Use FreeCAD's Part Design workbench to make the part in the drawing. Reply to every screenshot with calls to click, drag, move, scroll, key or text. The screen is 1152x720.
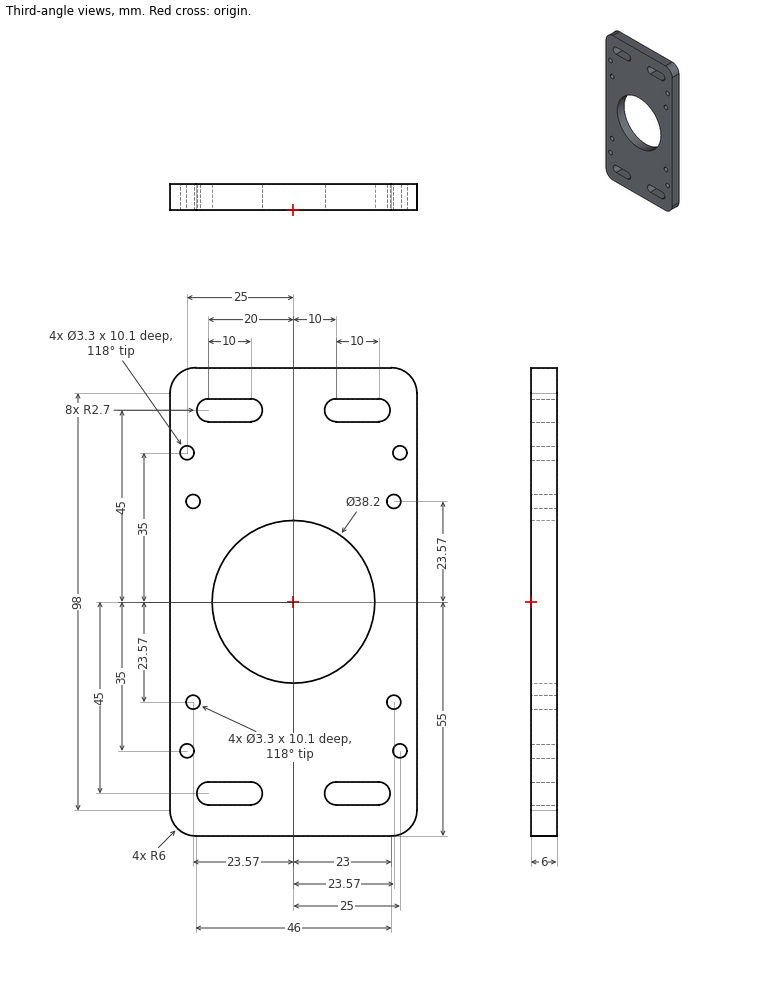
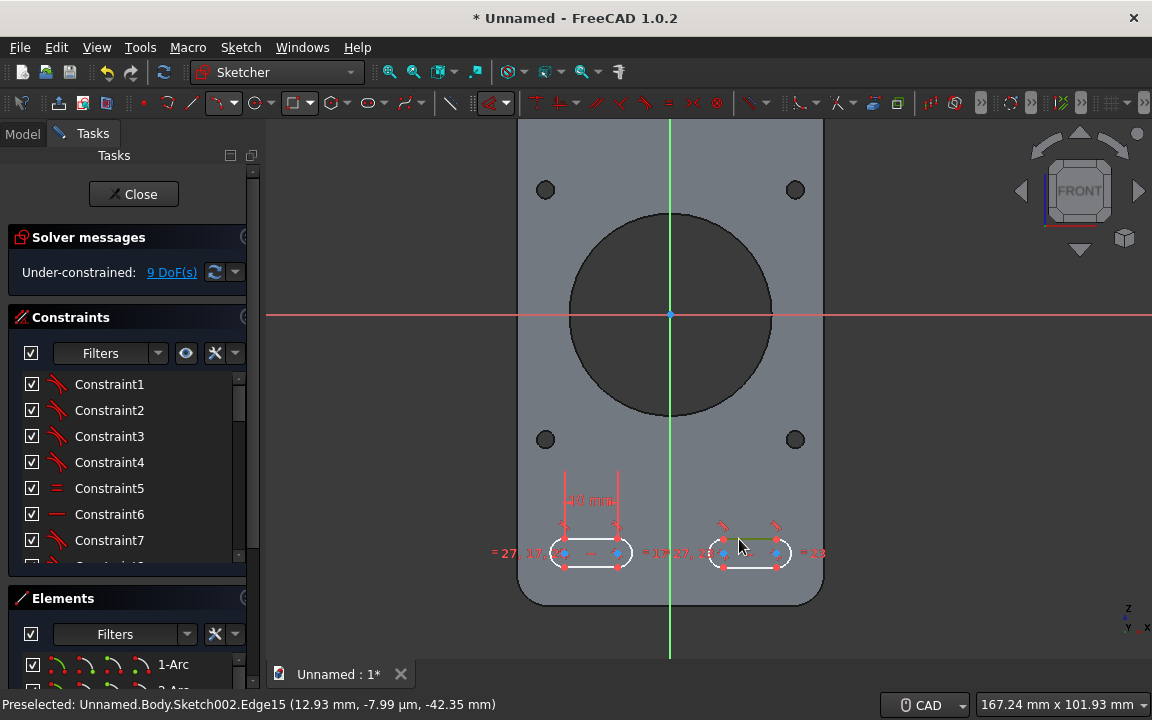
key(l)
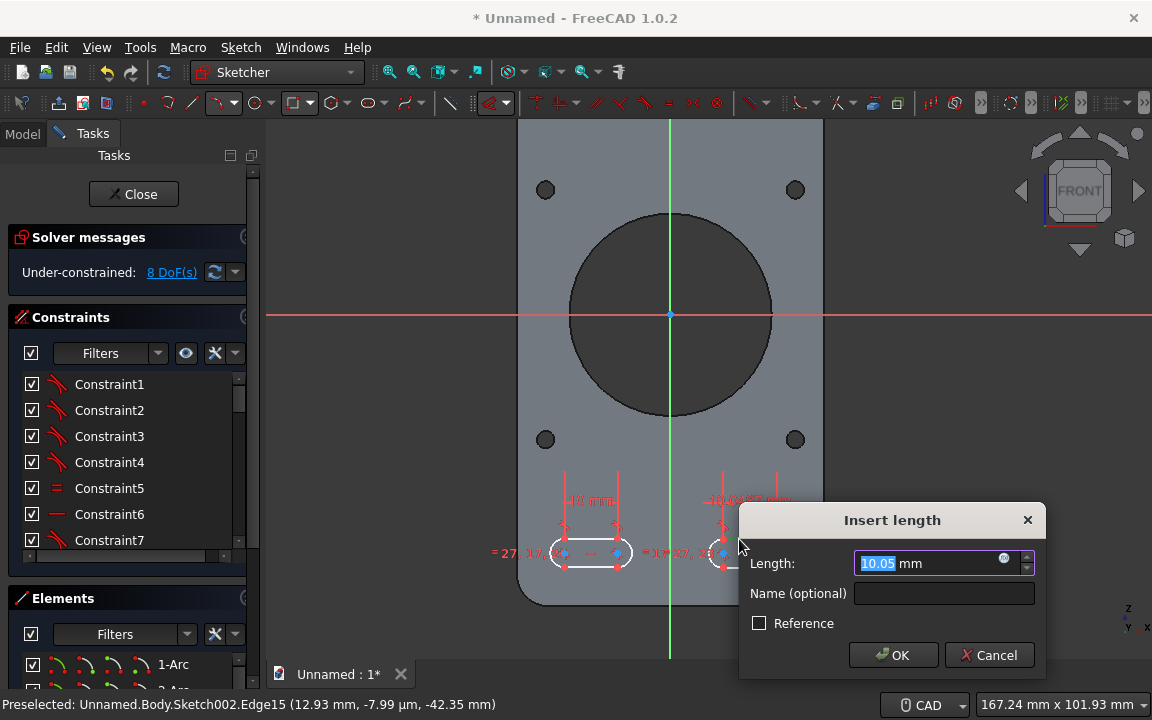
text(10)
key(Return)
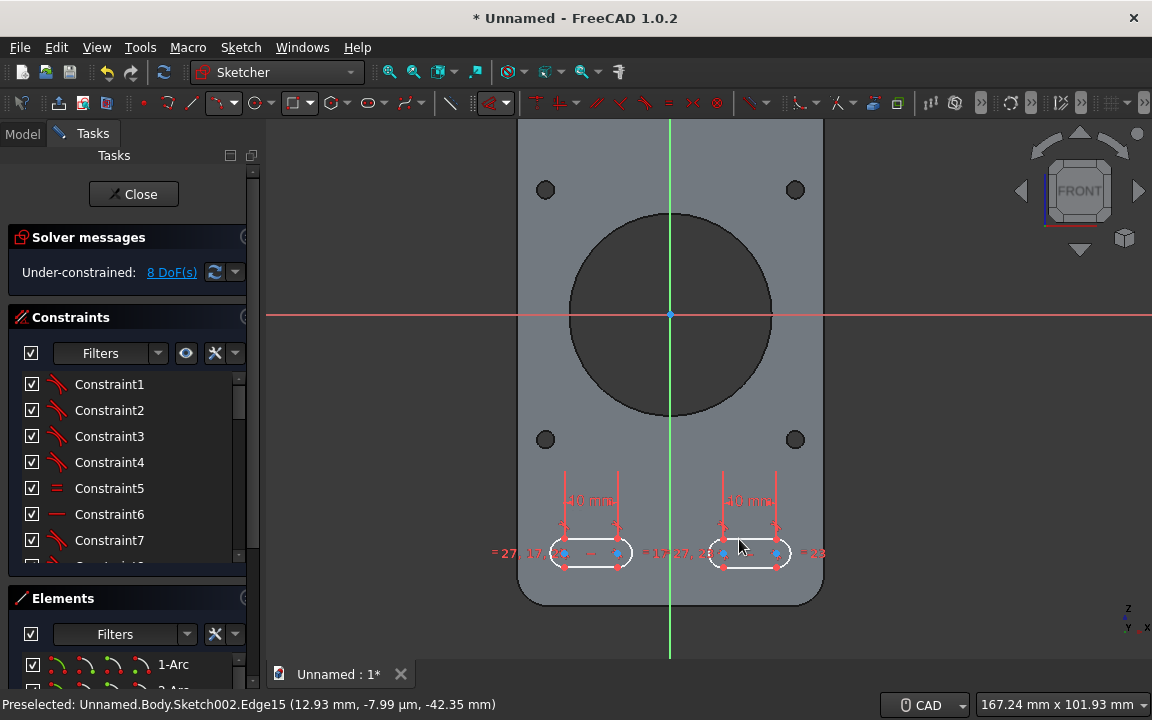
scroll(580, 540, down, 2)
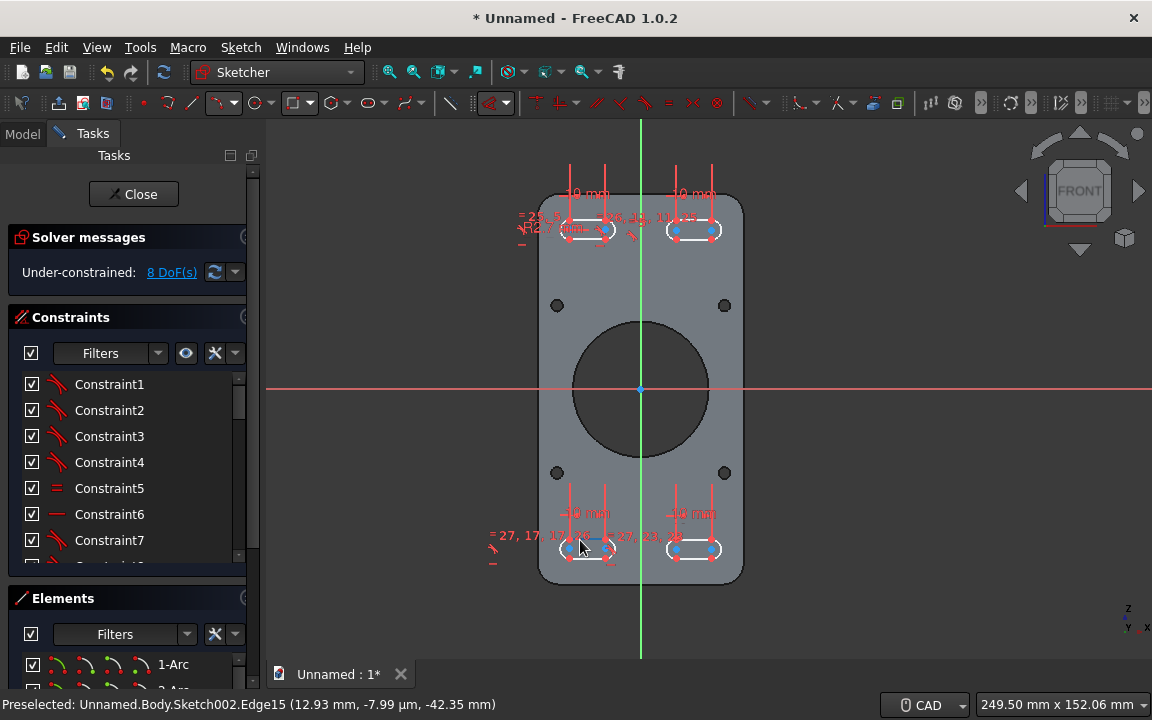
scroll(570, 220, up, 2)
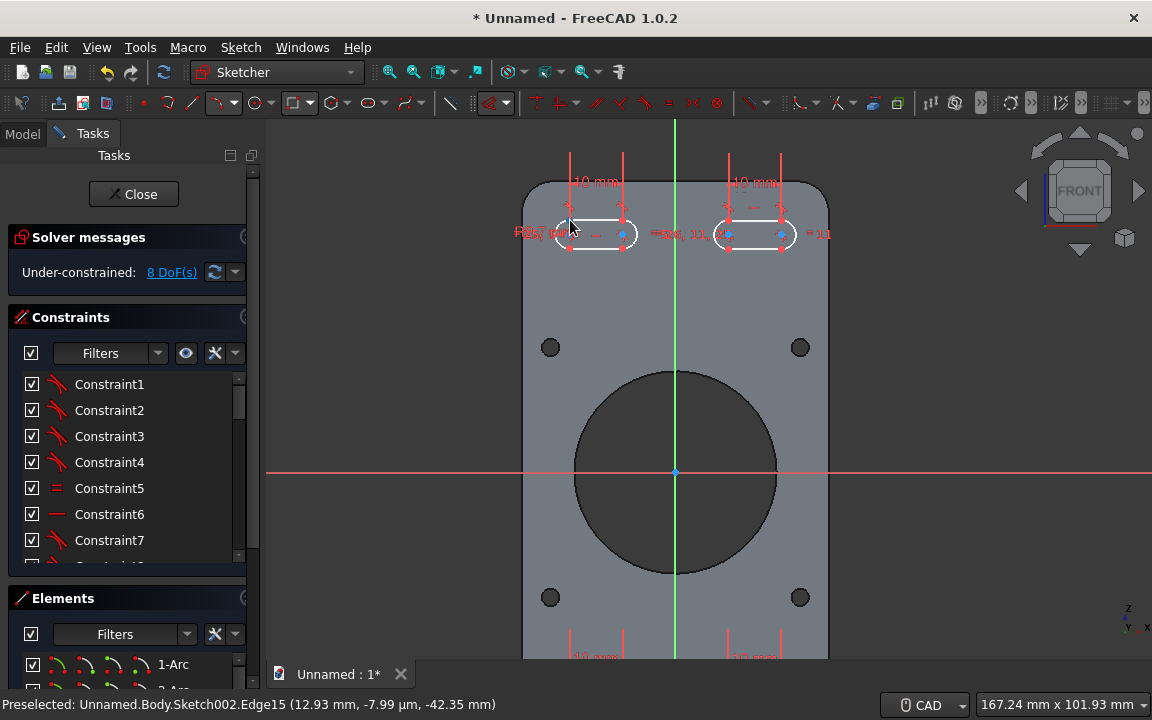
click(570, 220)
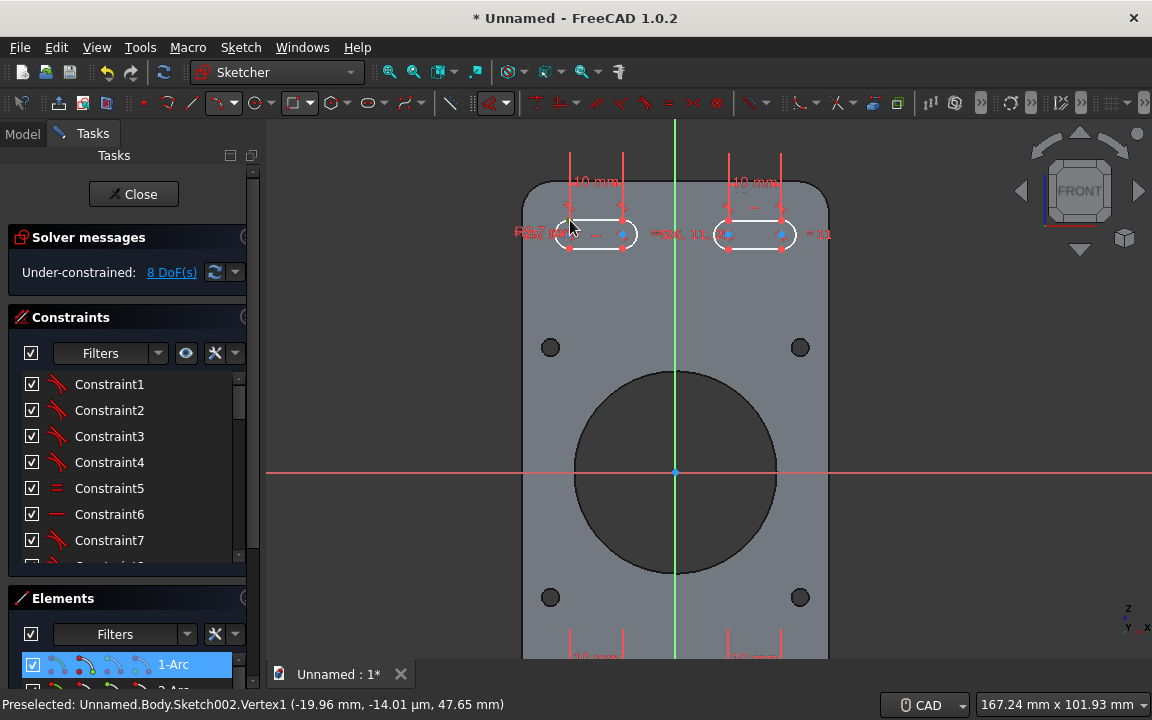
click(508, 104)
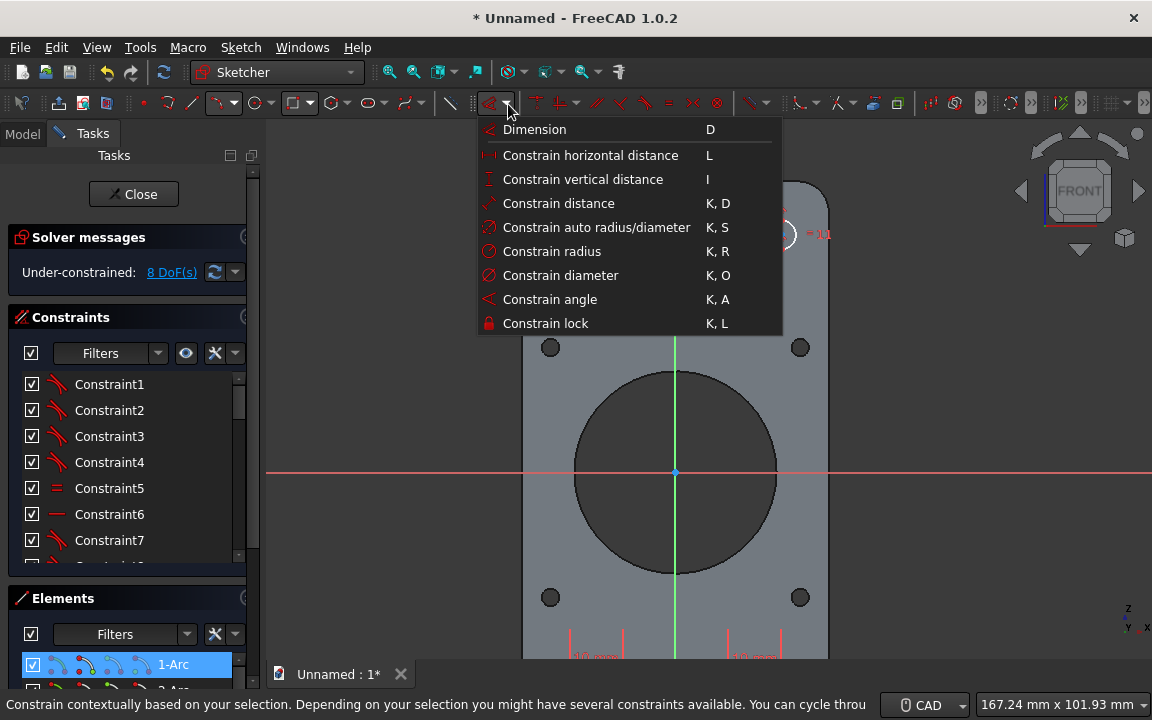
click(630, 155)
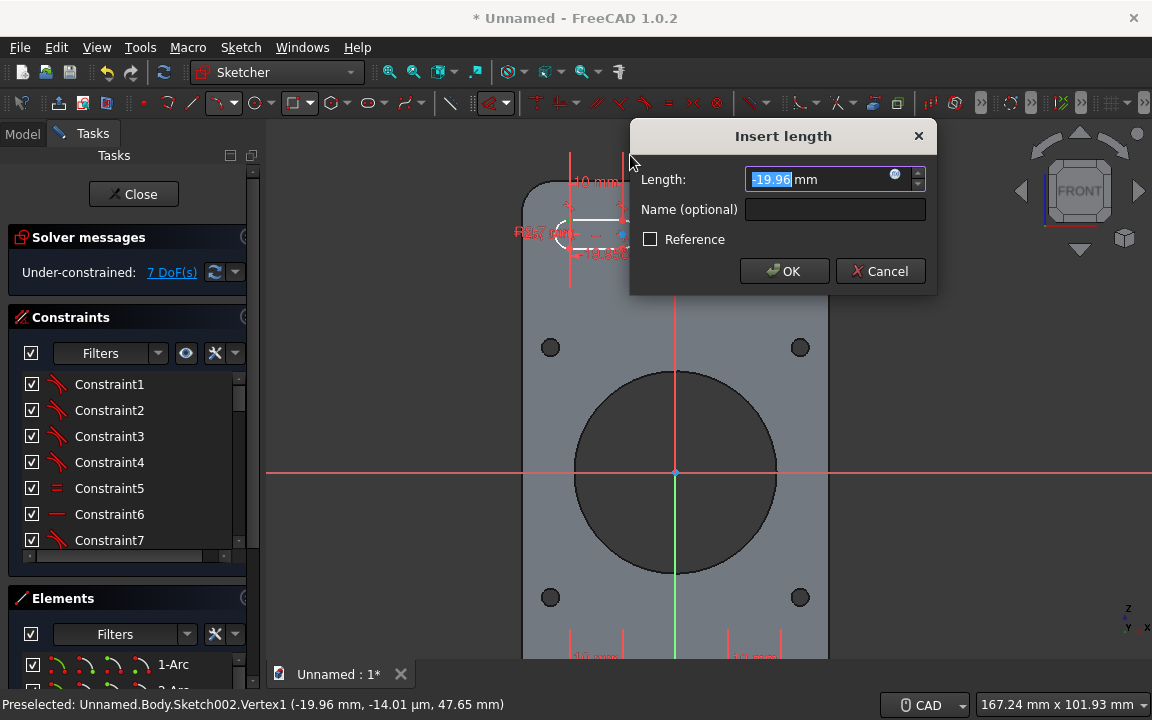
text(-20)
key(Return)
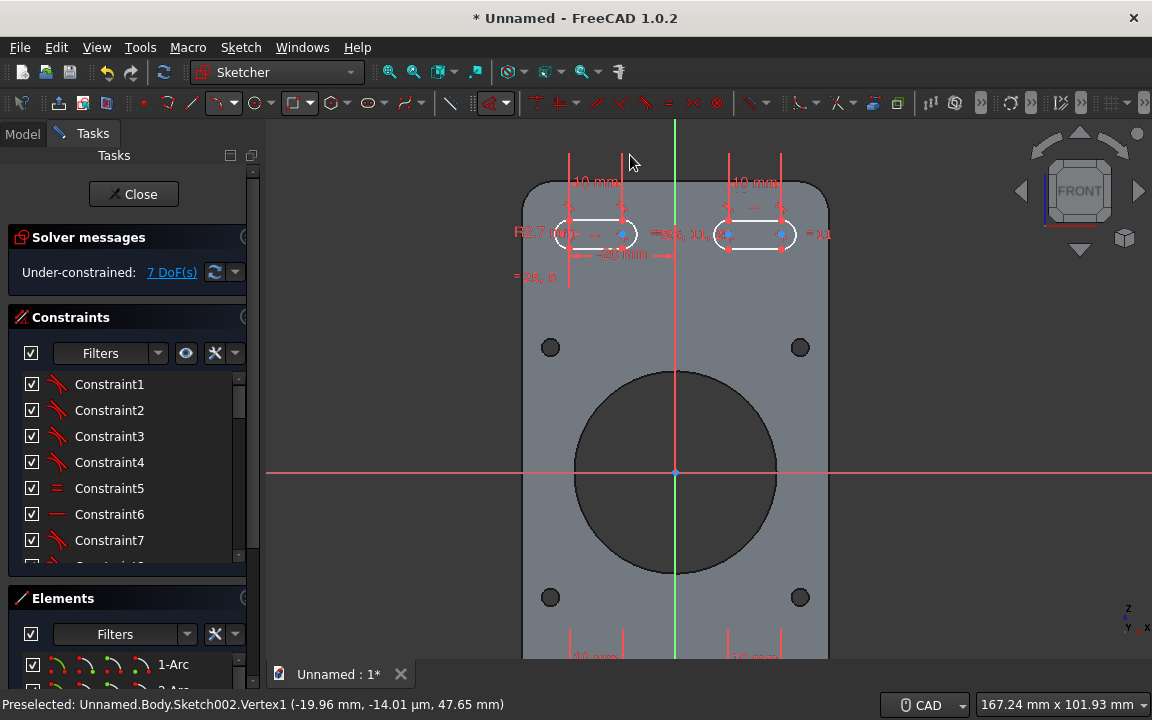
click(729, 221)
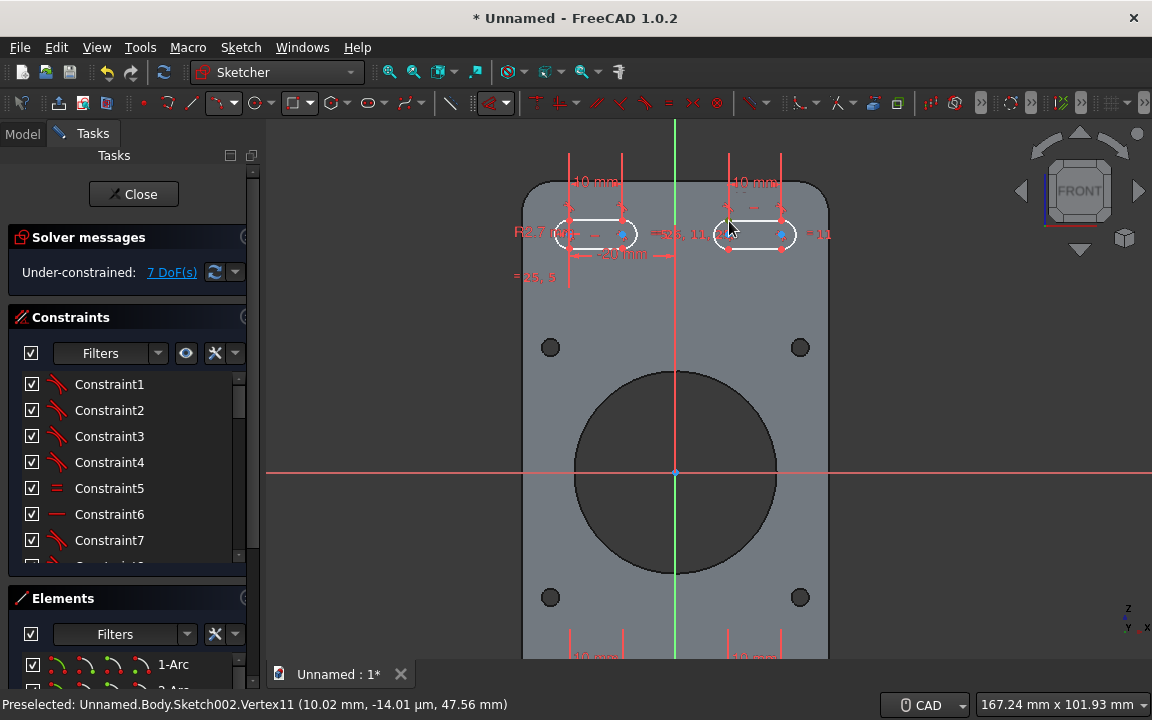
click(508, 104)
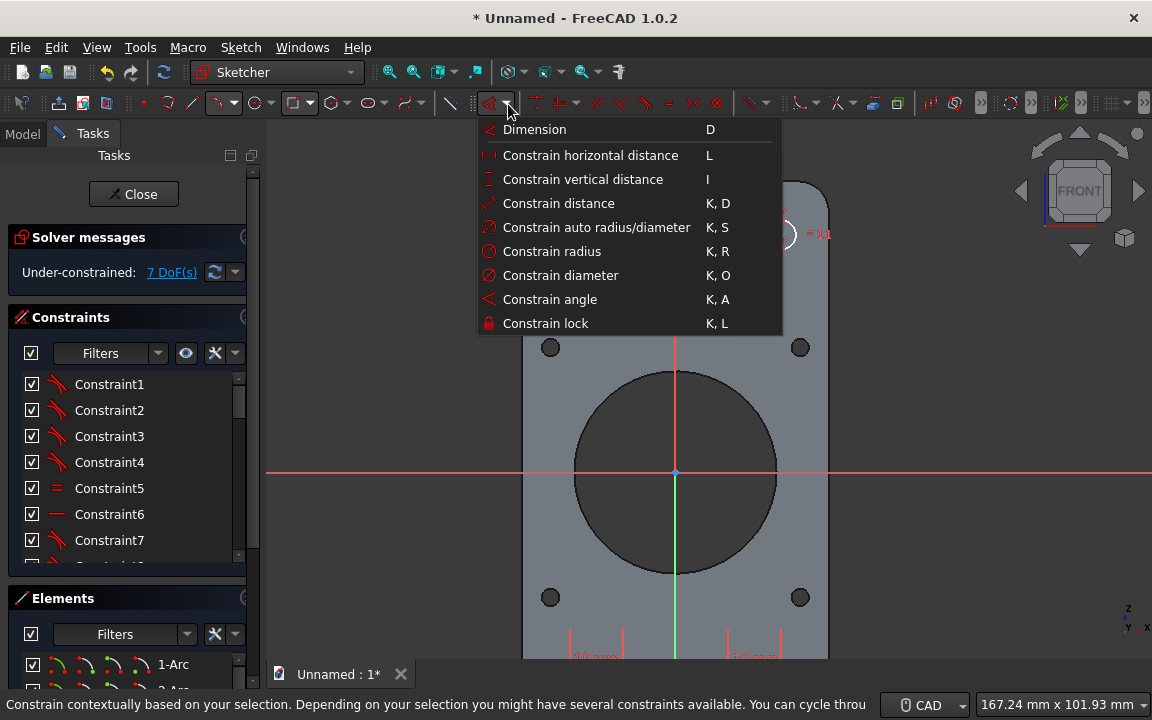
click(630, 155)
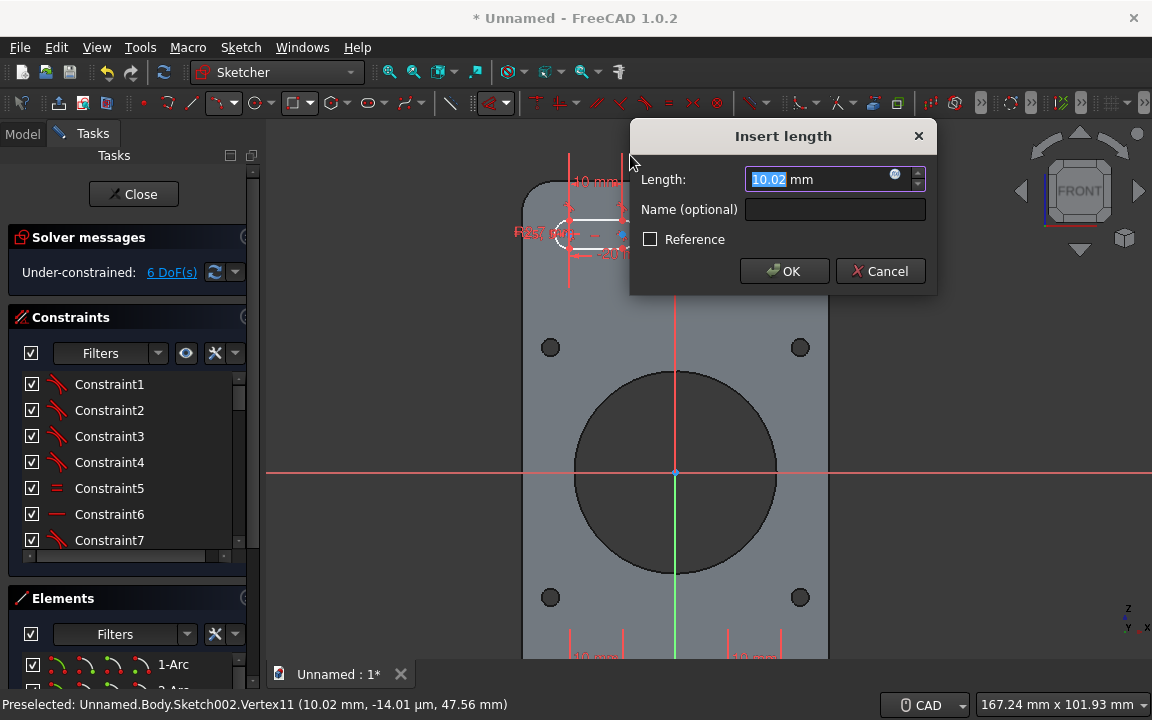
text(10)
key(Return)